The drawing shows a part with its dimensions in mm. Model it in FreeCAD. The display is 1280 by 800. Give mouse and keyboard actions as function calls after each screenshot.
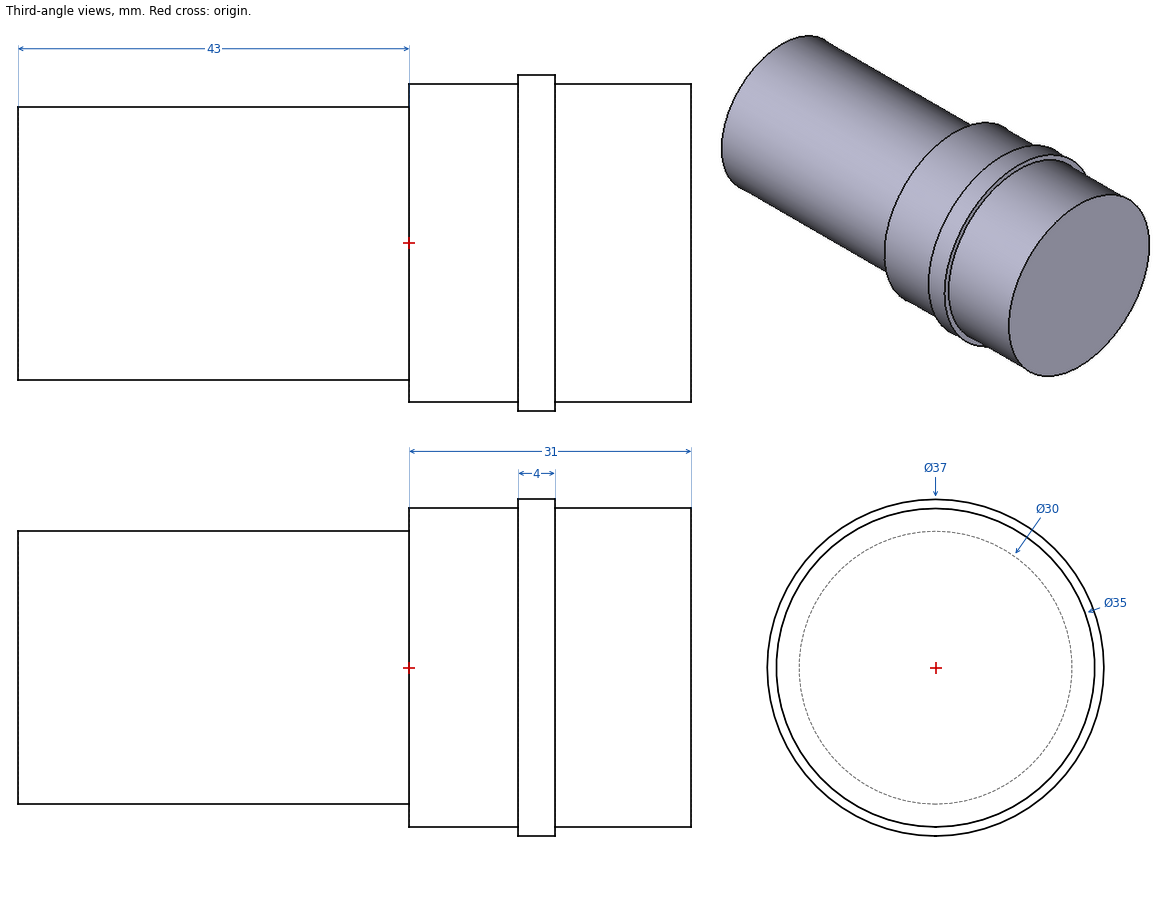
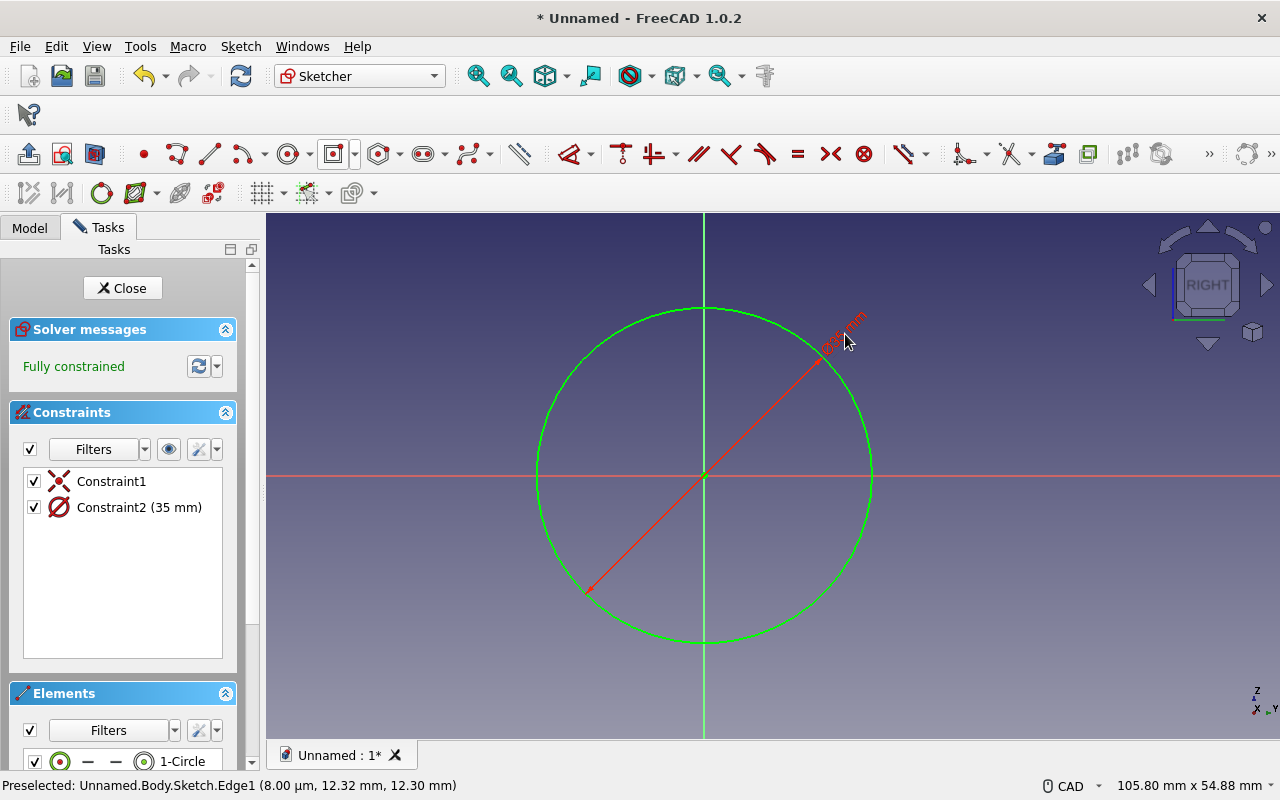
click(123, 288)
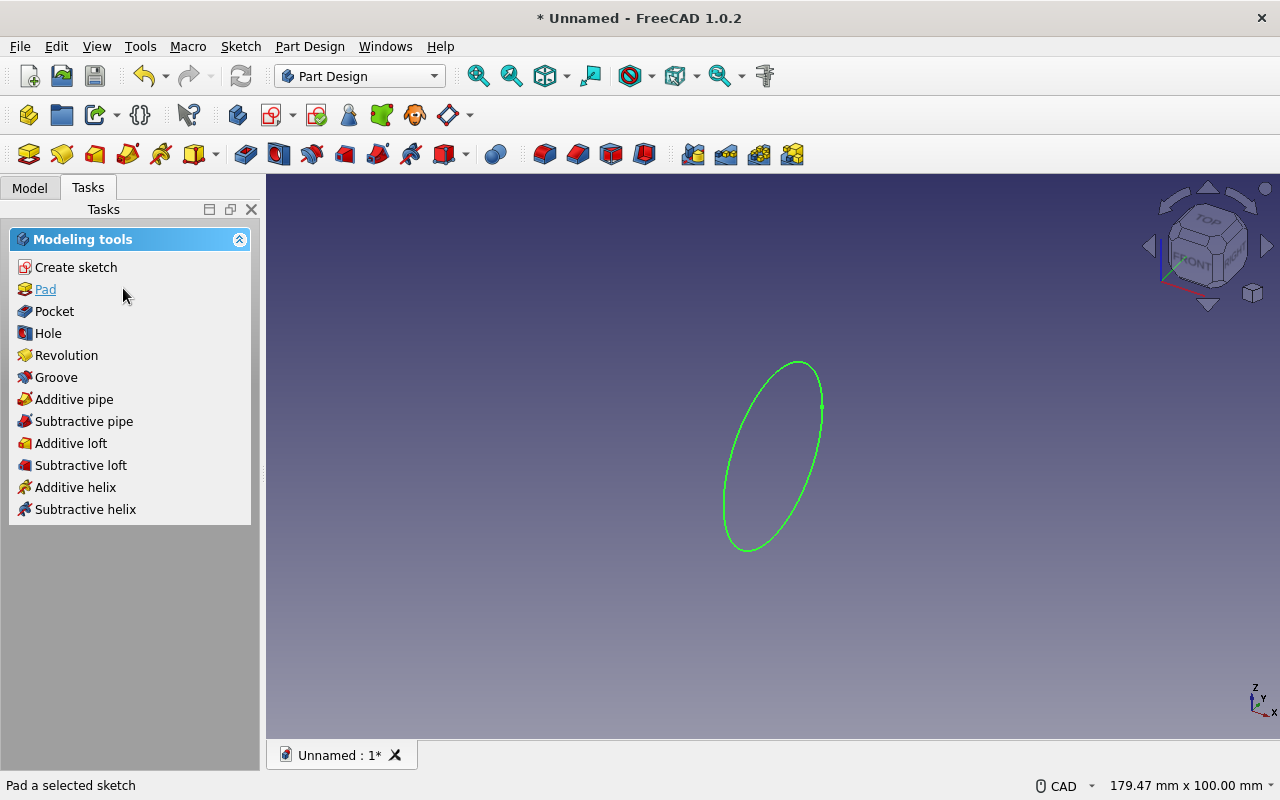
click(29, 154)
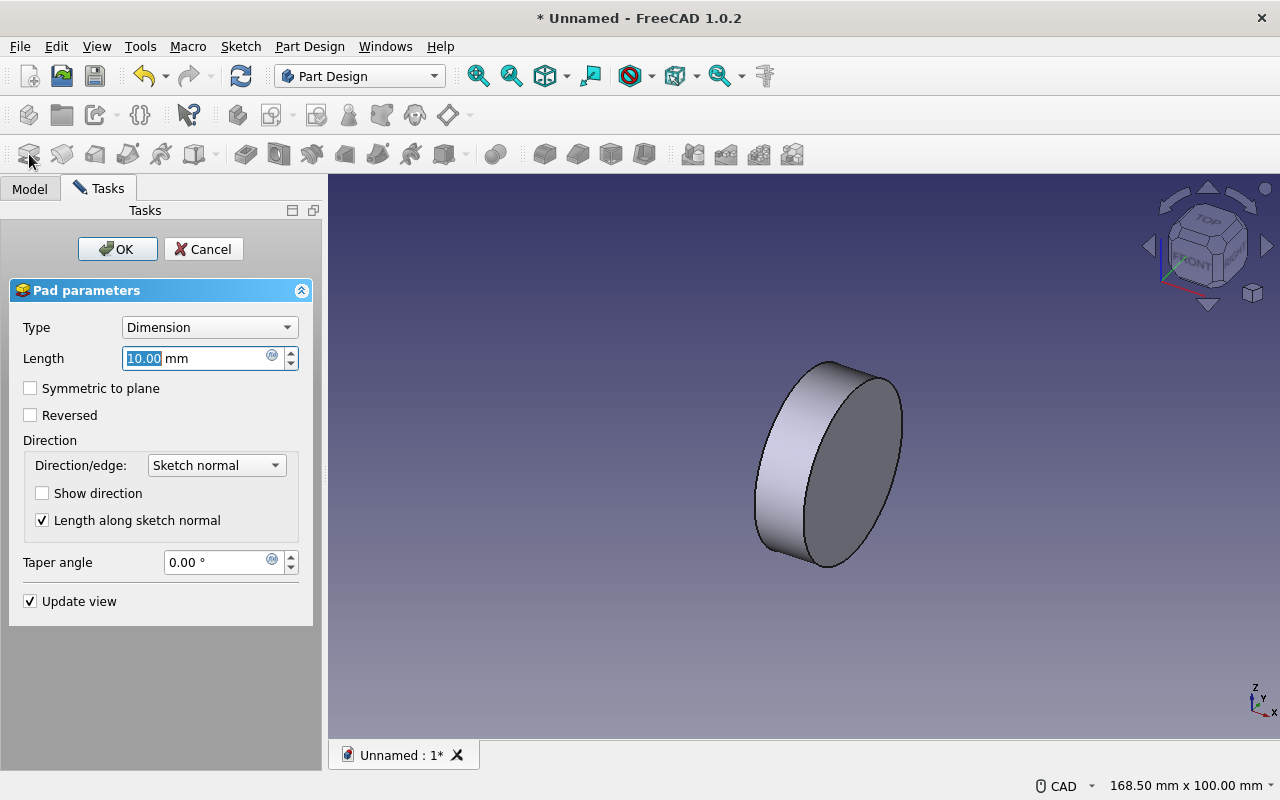
text(31)
key(Tab)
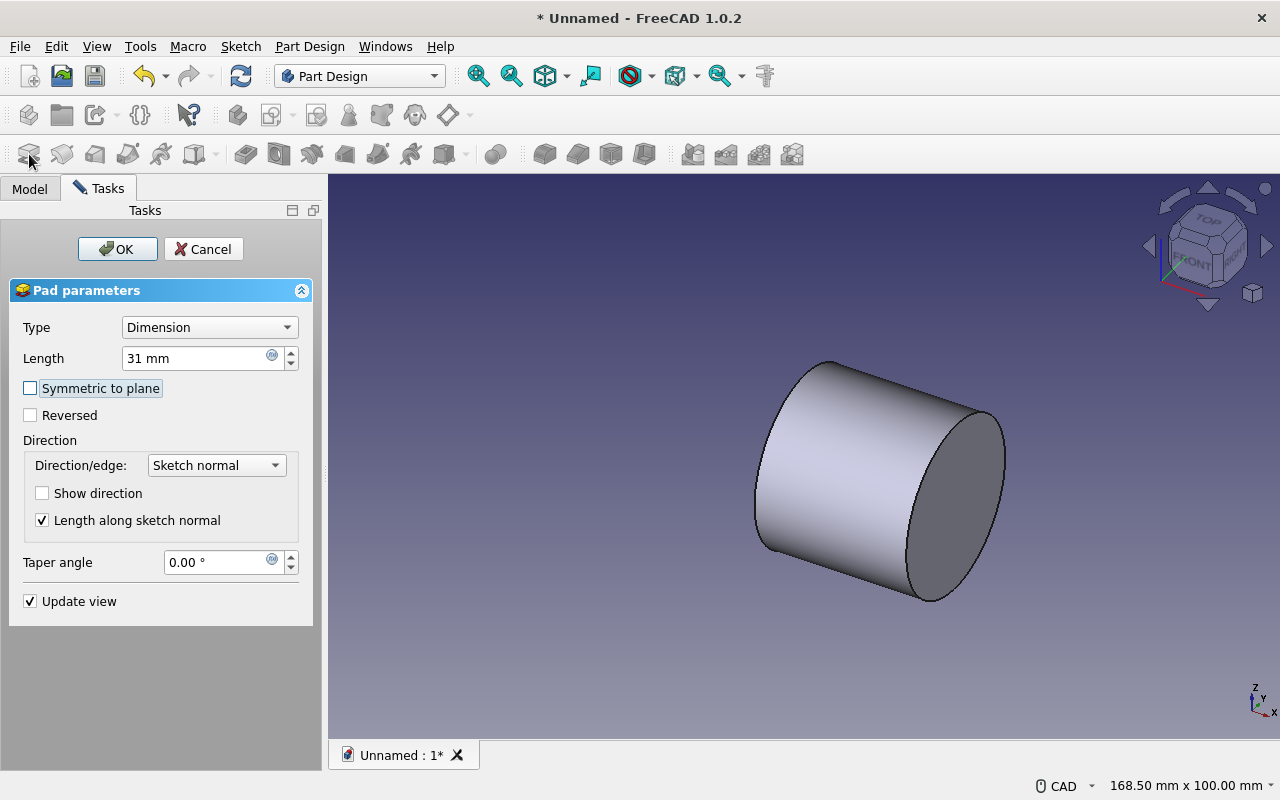
click(118, 249)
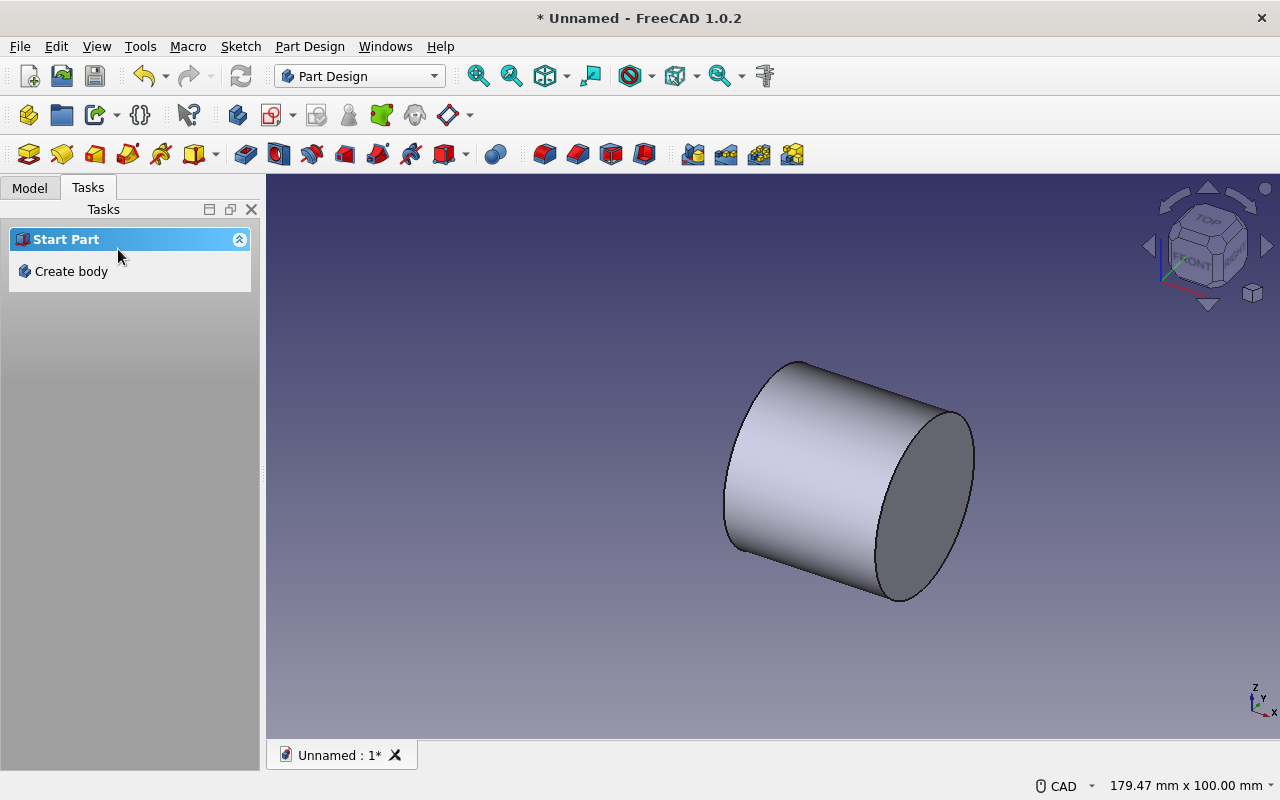
key(6)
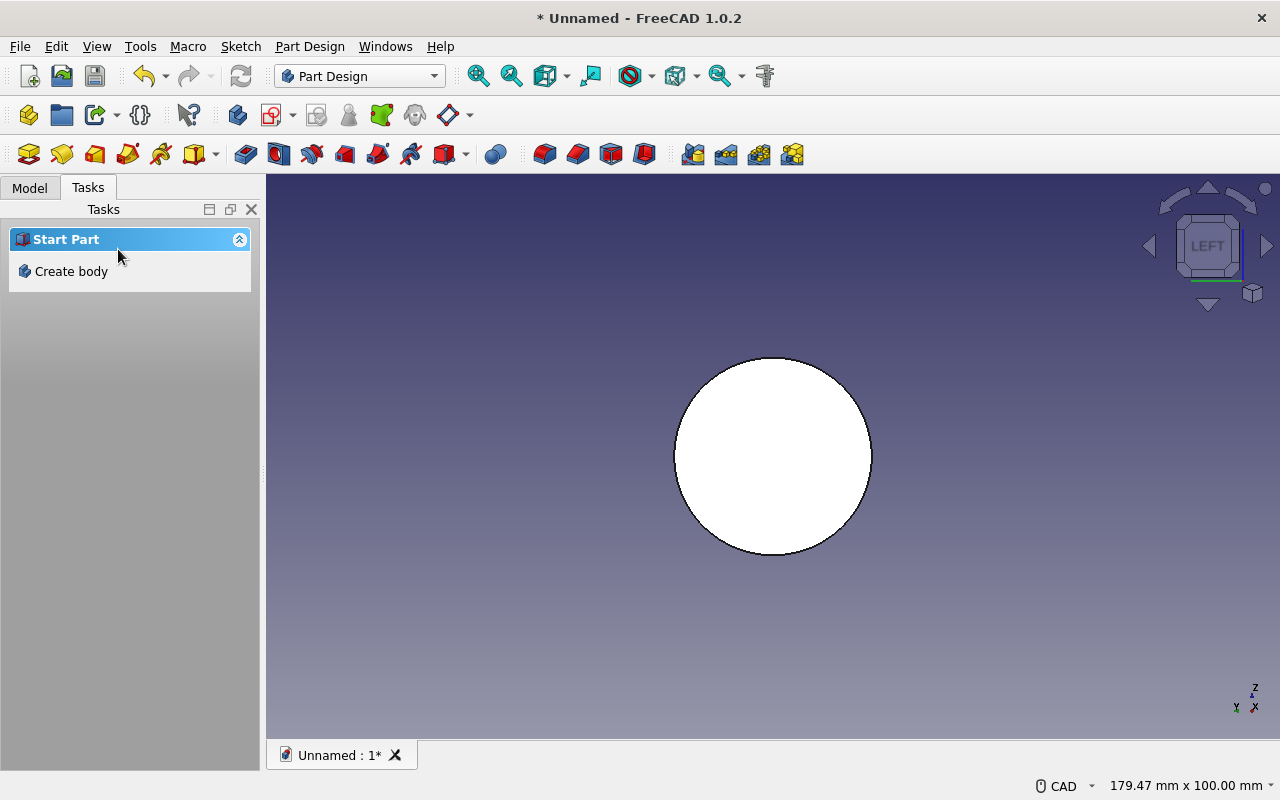
key(v)
key(f)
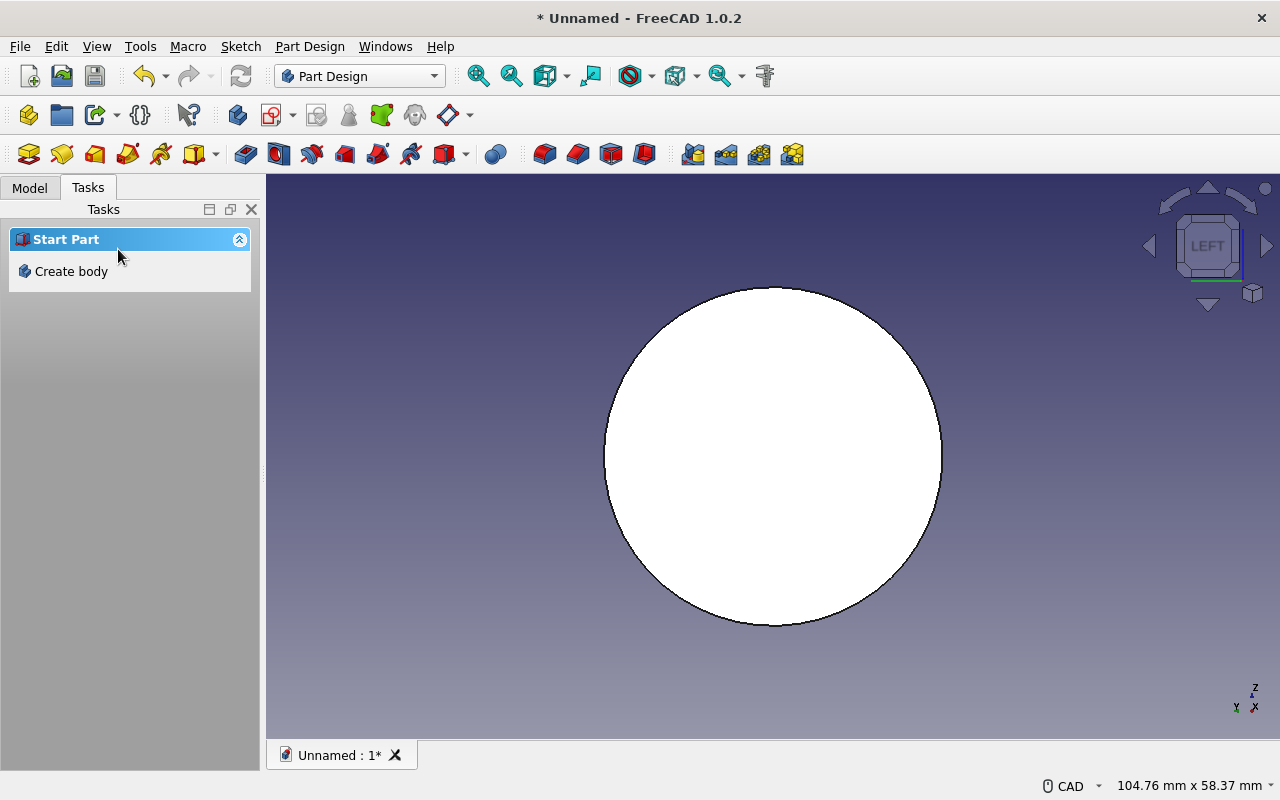
click(773, 455)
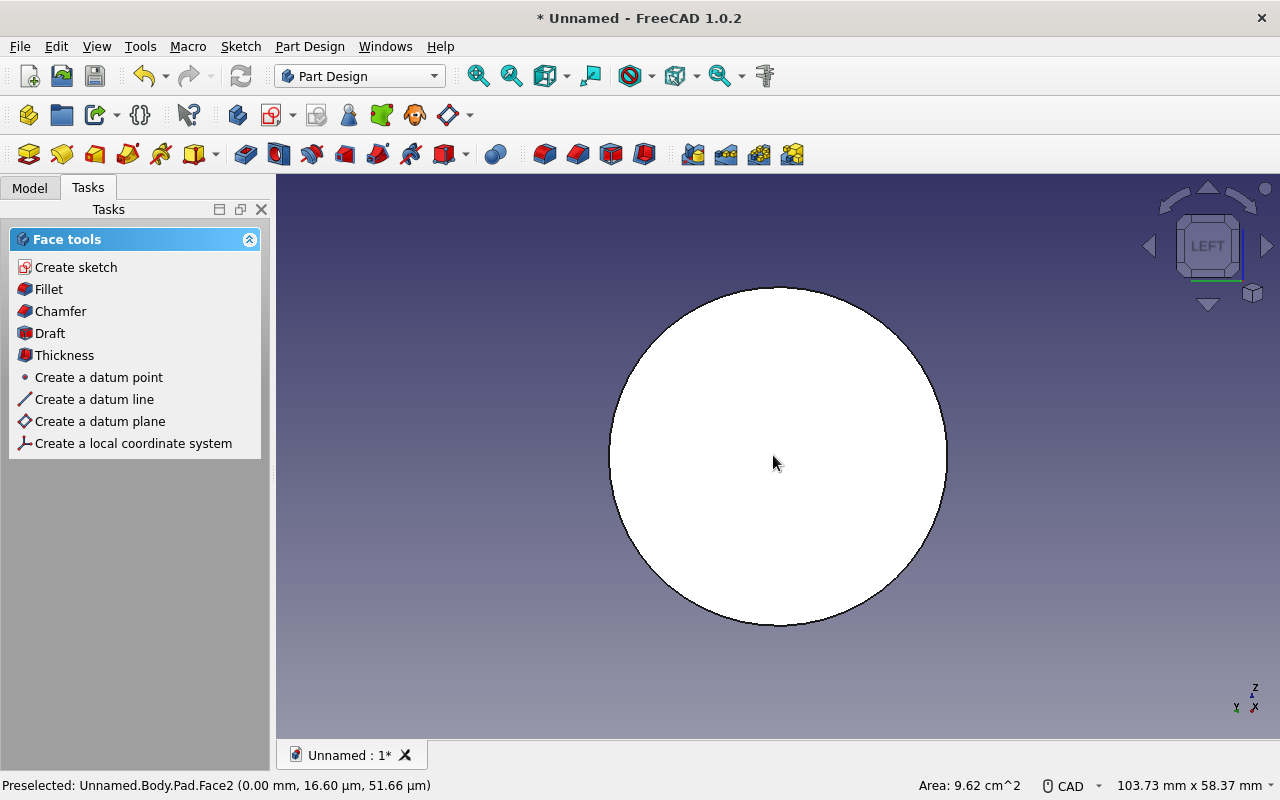
click(270, 116)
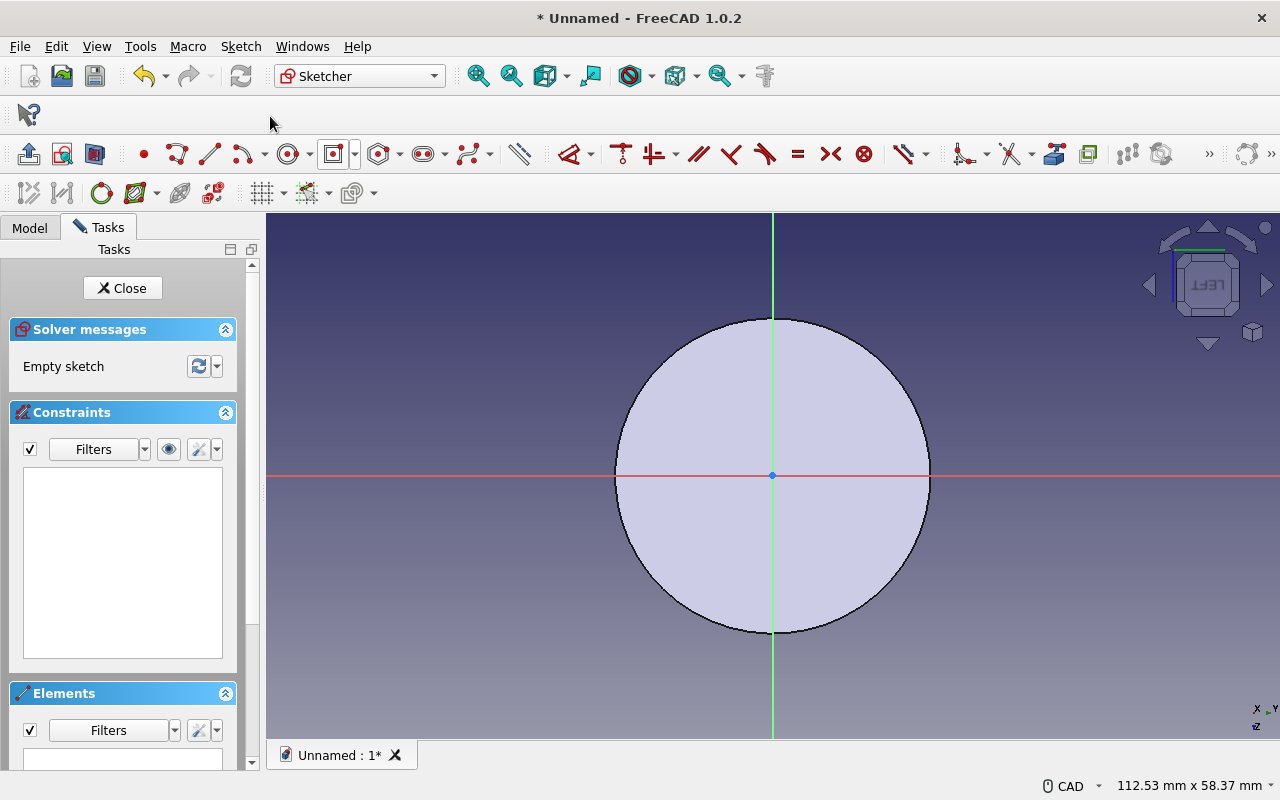
key(g)
key(c)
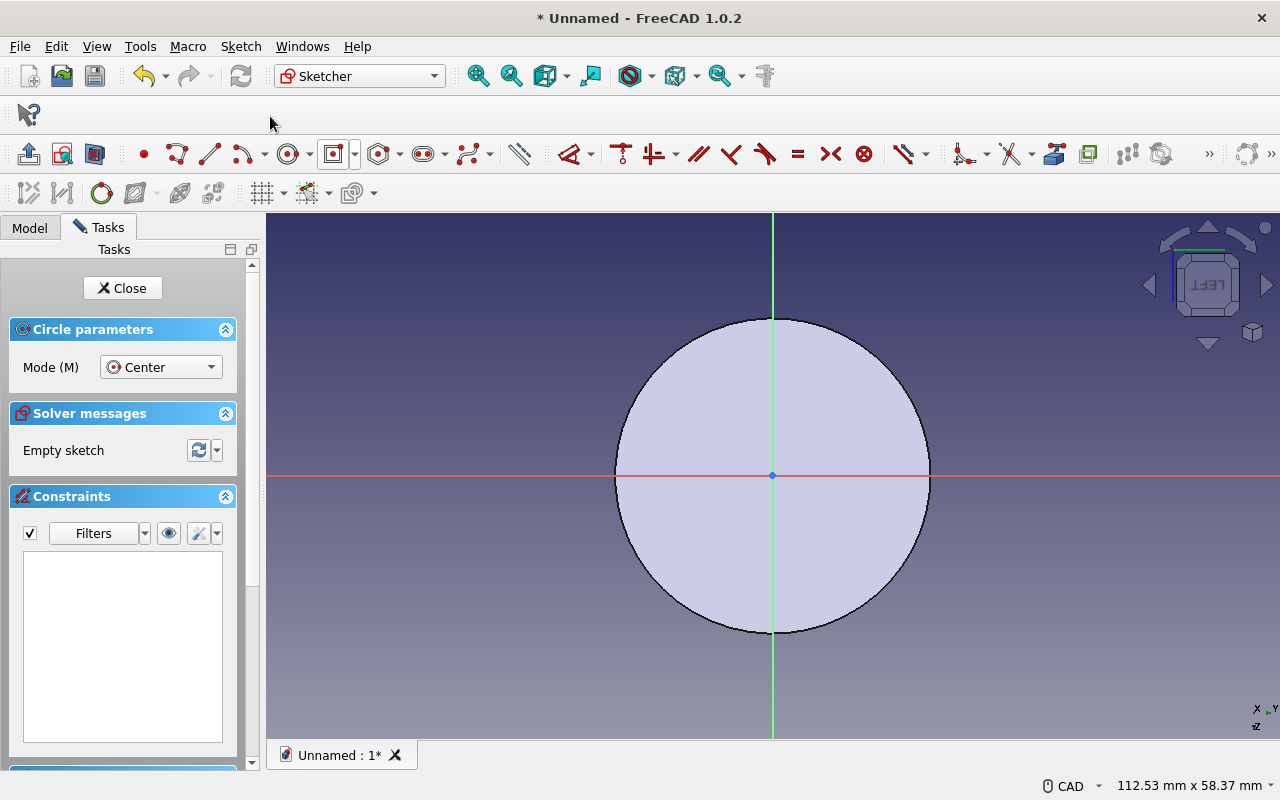
click(773, 476)
click(868, 380)
key(Escape)